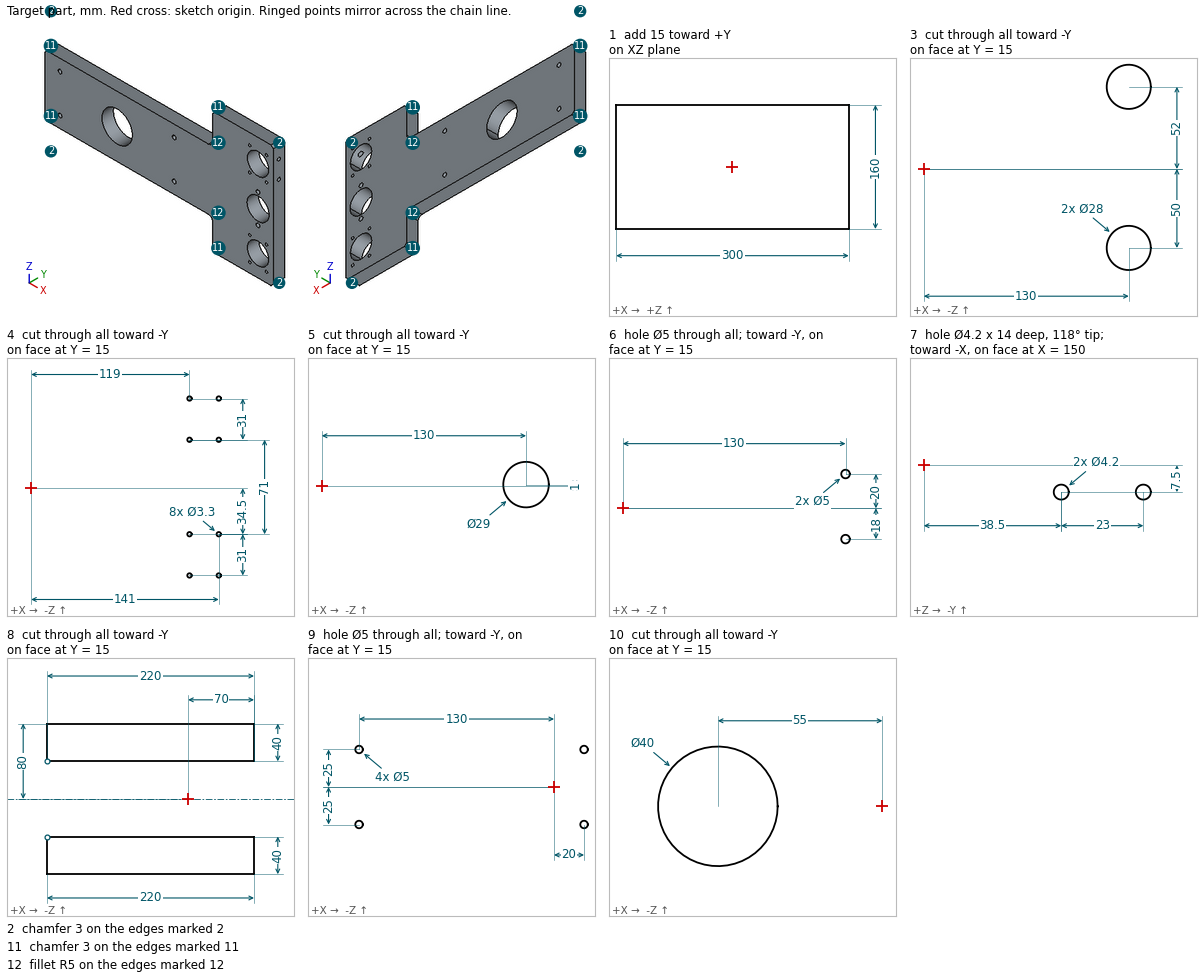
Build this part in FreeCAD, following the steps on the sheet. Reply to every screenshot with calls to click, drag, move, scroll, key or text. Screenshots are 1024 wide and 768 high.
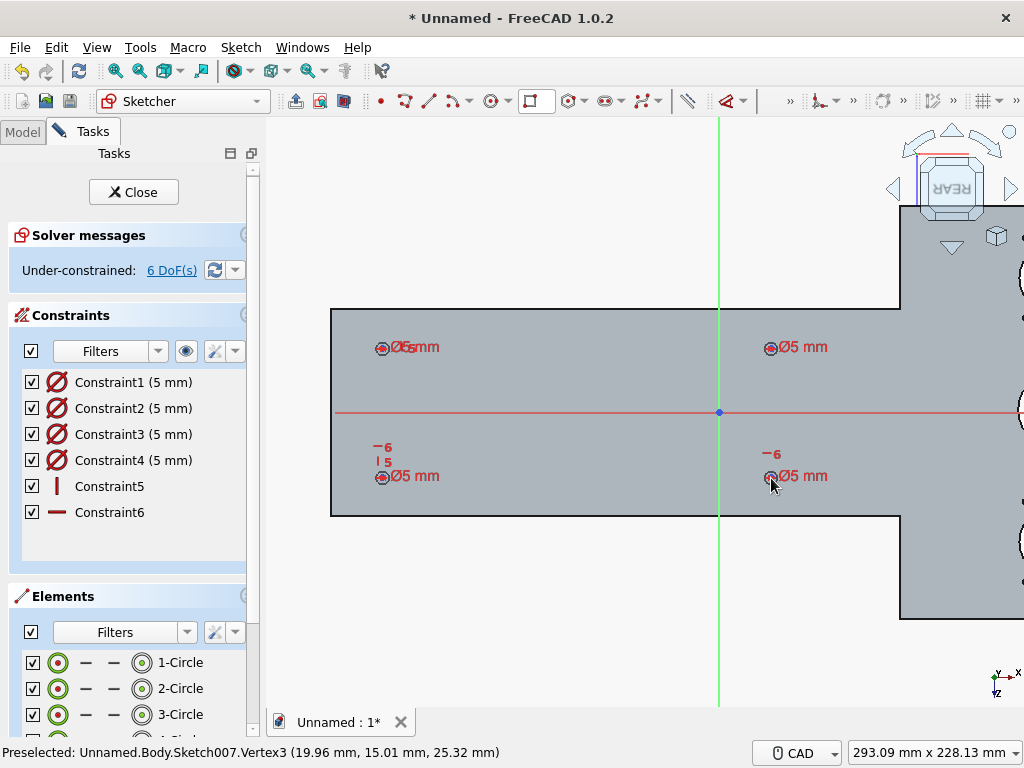
click(771, 478)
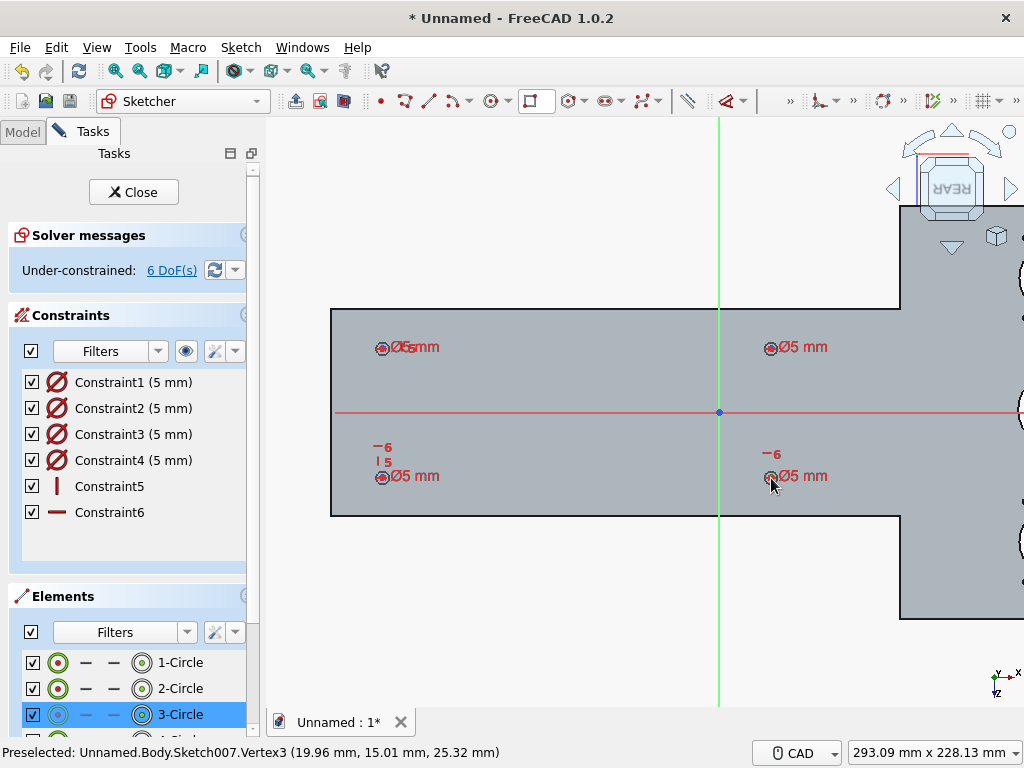
click(771, 349)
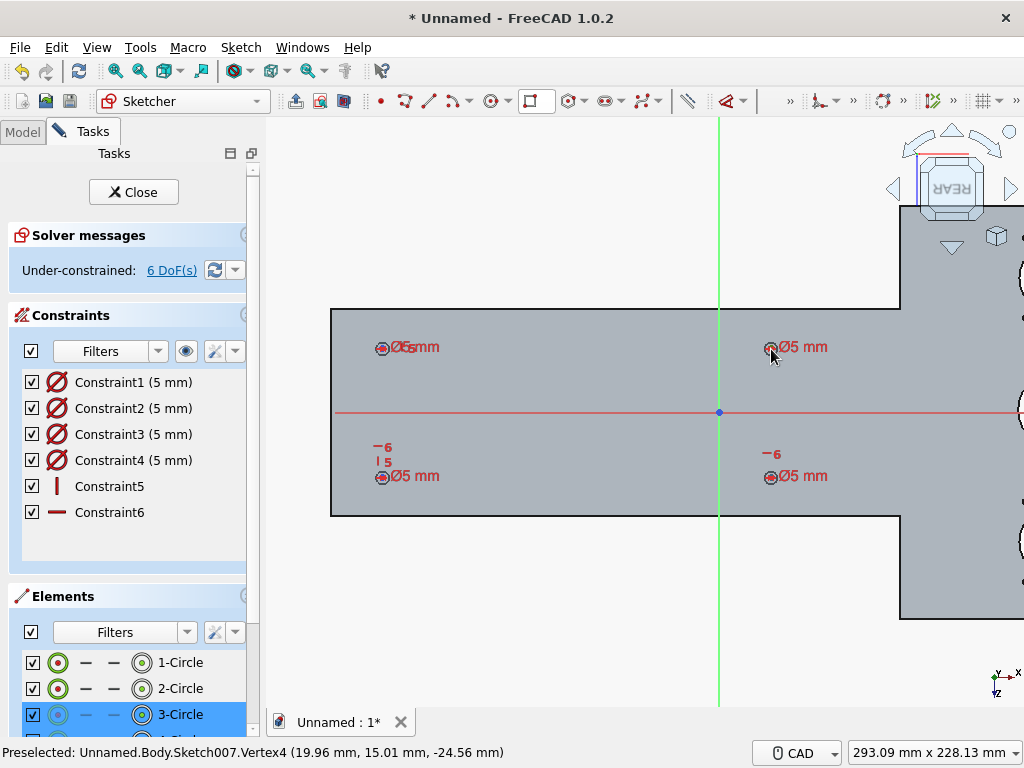
key(v)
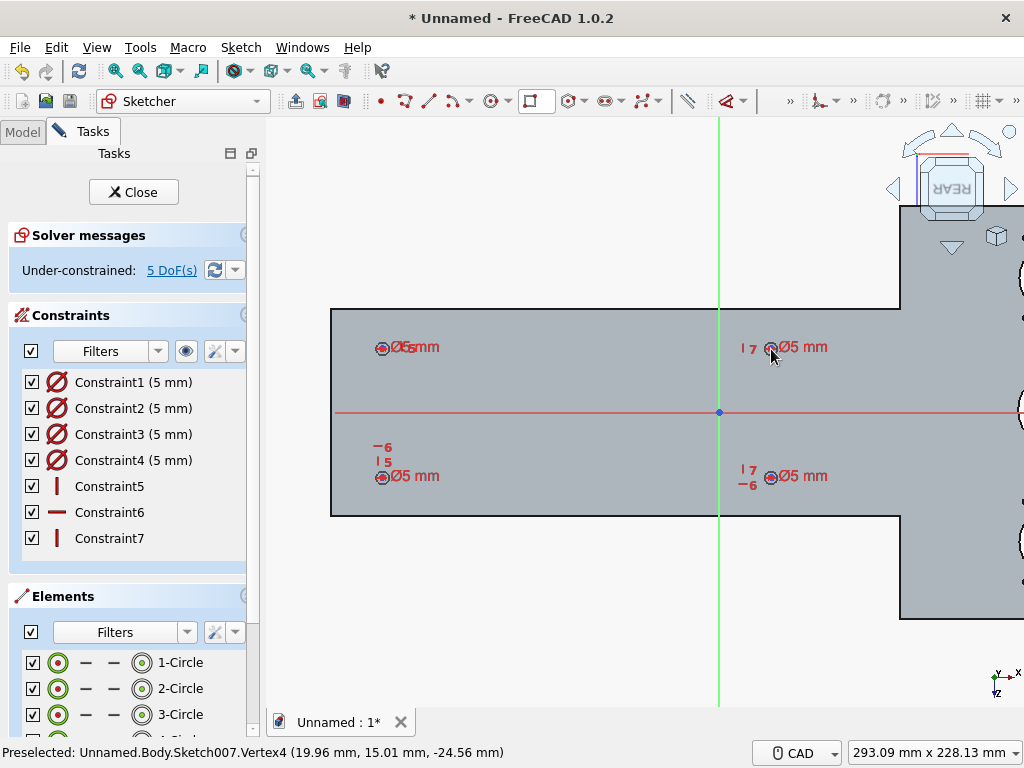
click(383, 349)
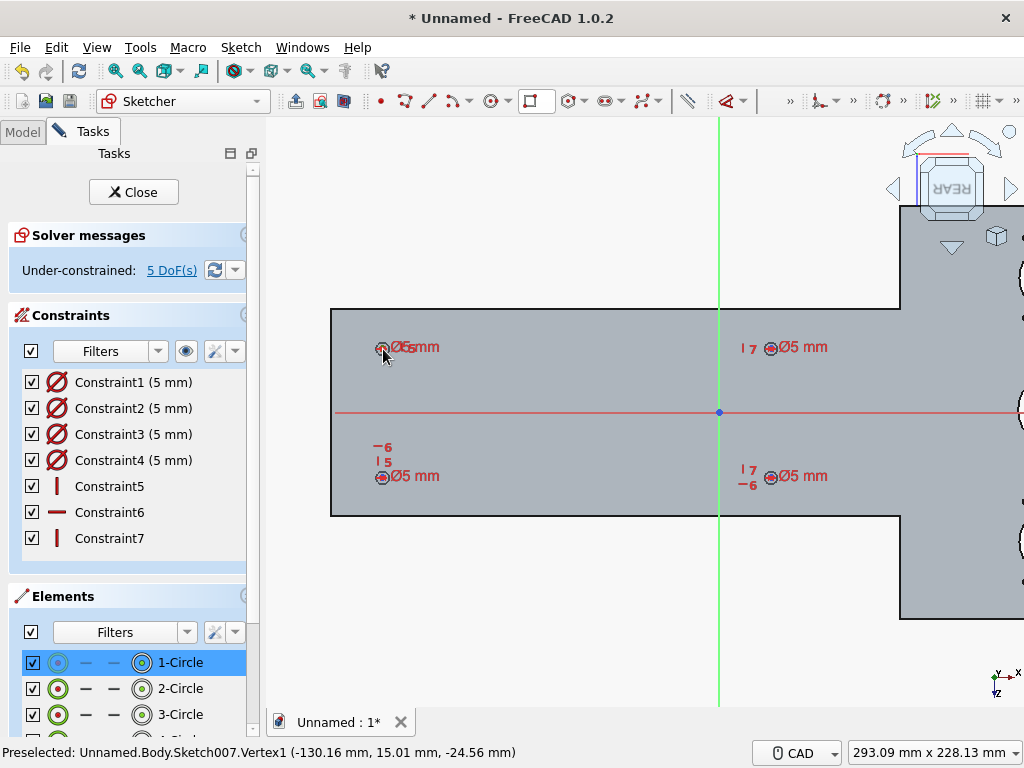
click(771, 349)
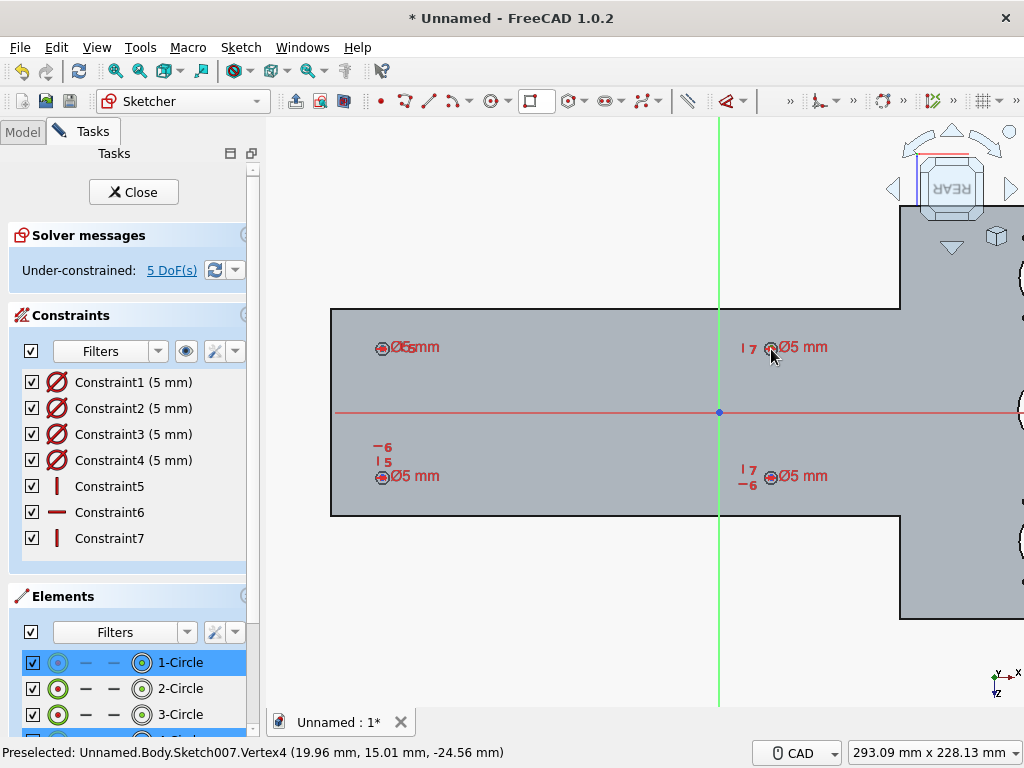
key(h)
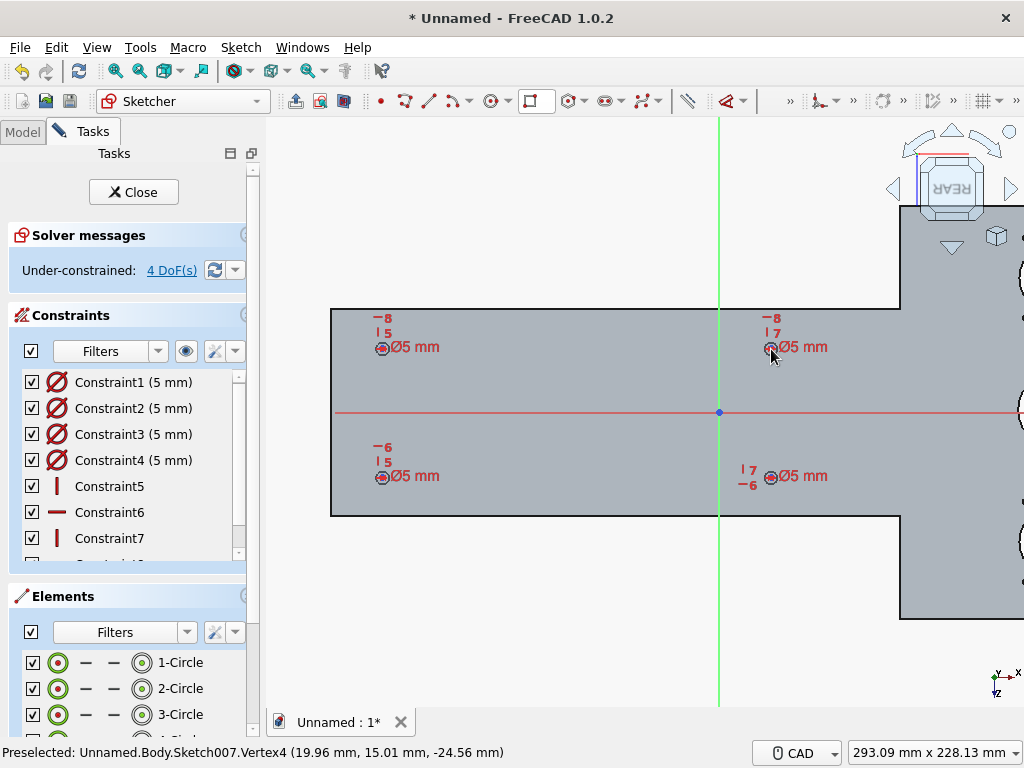
click(726, 102)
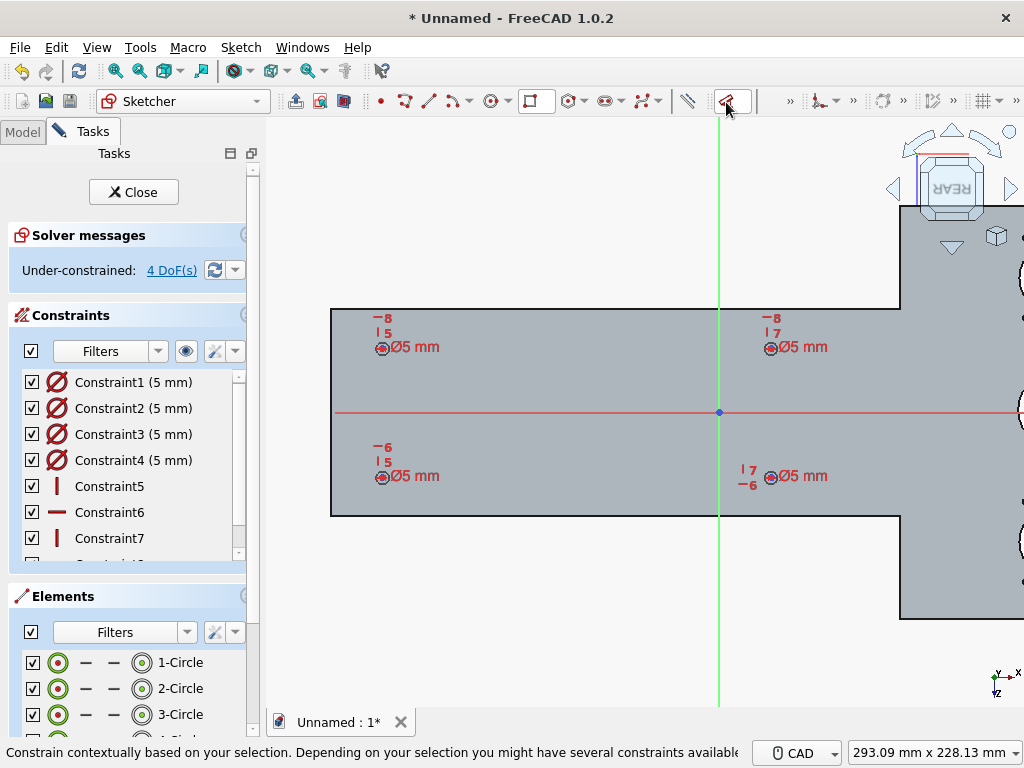
click(383, 349)
click(349, 381)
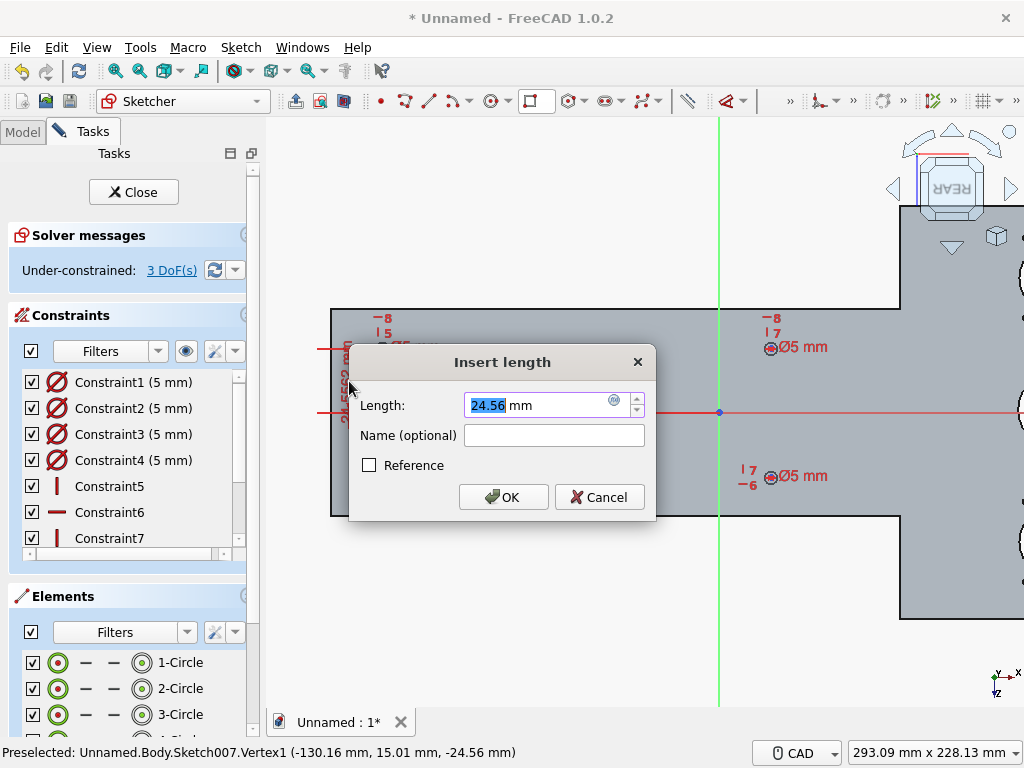
text(25)
key(Return)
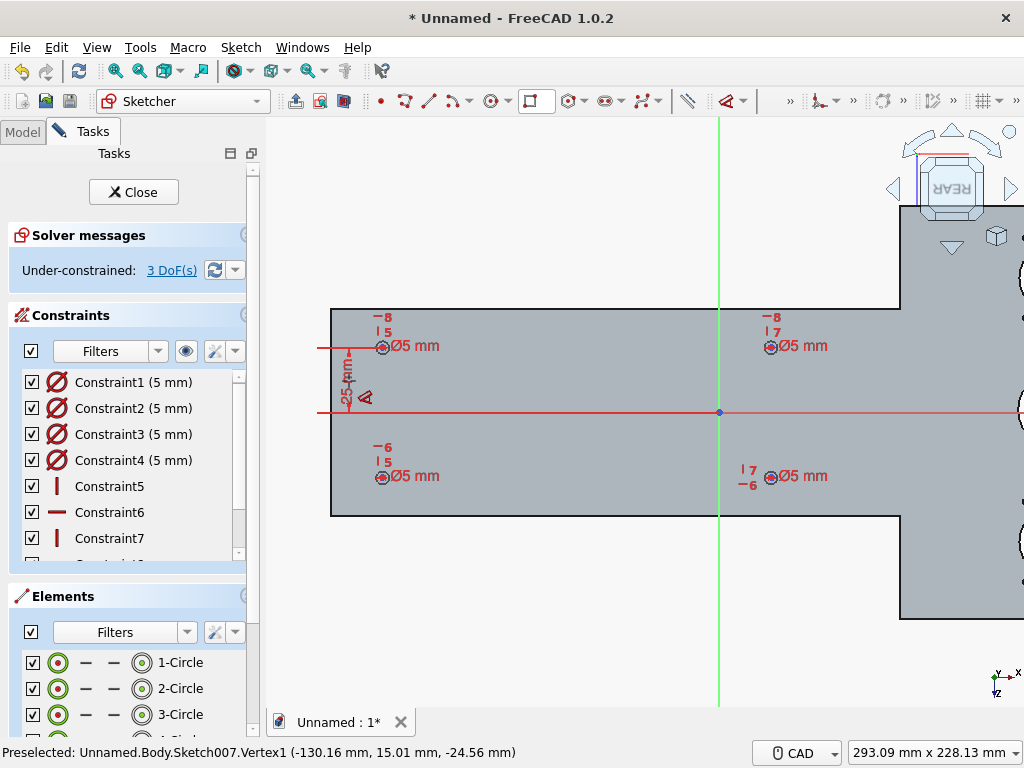
click(383, 478)
click(349, 445)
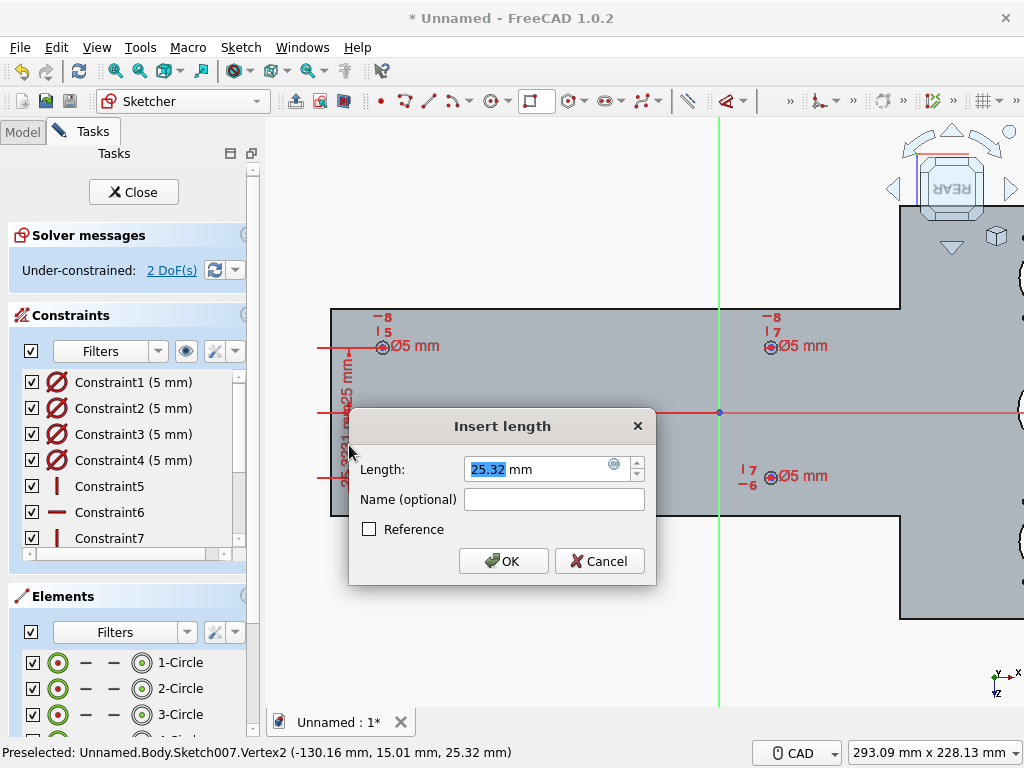
text(25)
key(Return)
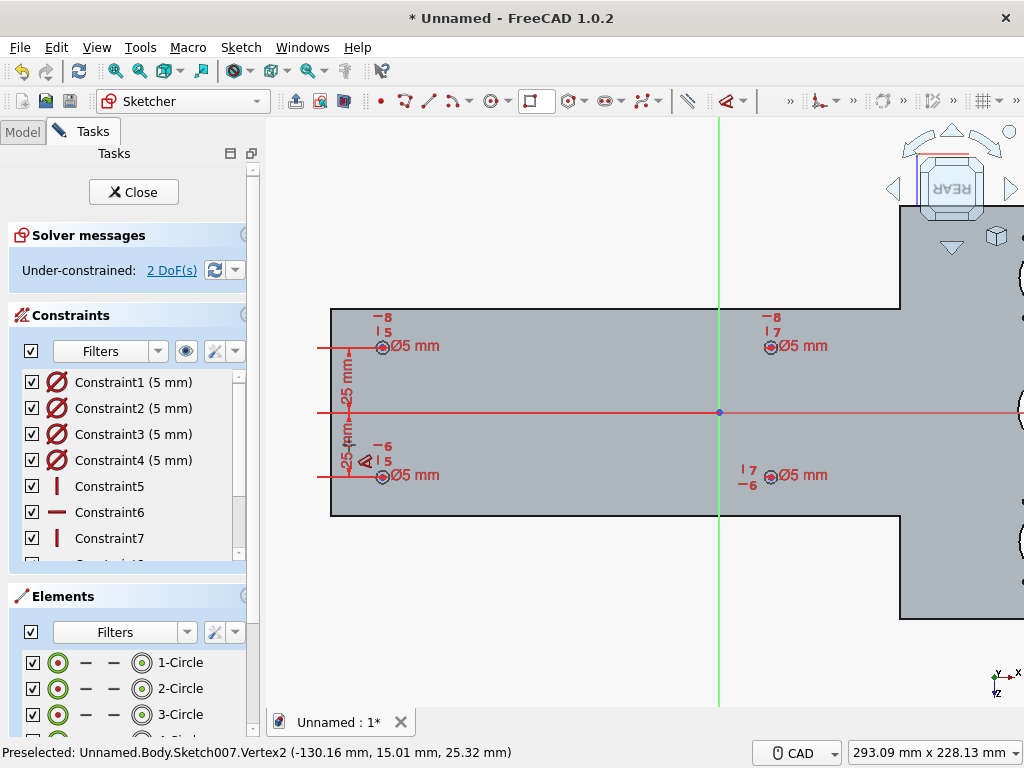
click(771, 477)
click(745, 511)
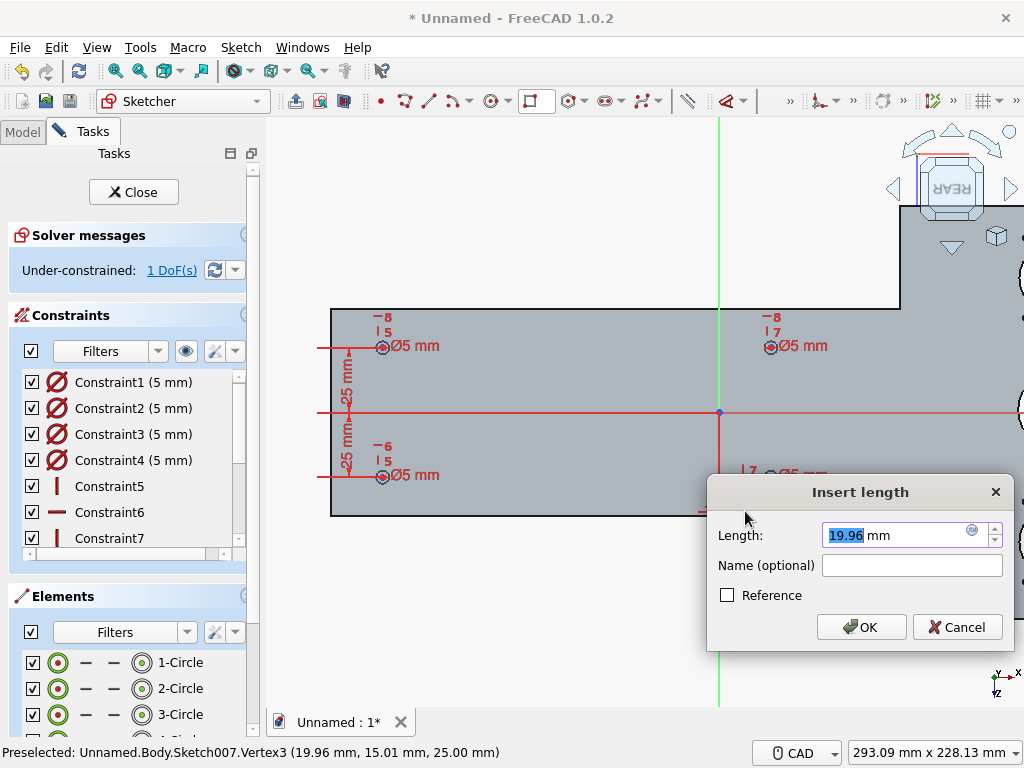
text(20)
key(Return)